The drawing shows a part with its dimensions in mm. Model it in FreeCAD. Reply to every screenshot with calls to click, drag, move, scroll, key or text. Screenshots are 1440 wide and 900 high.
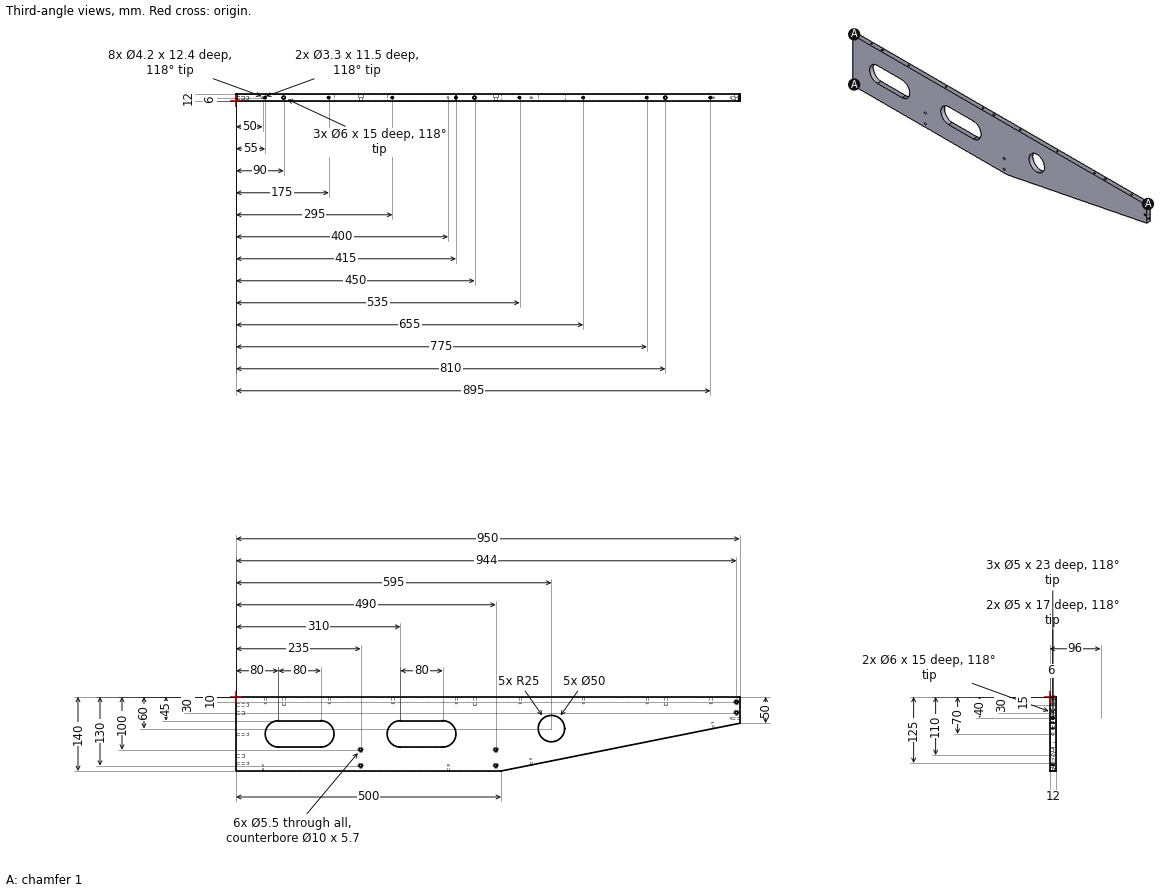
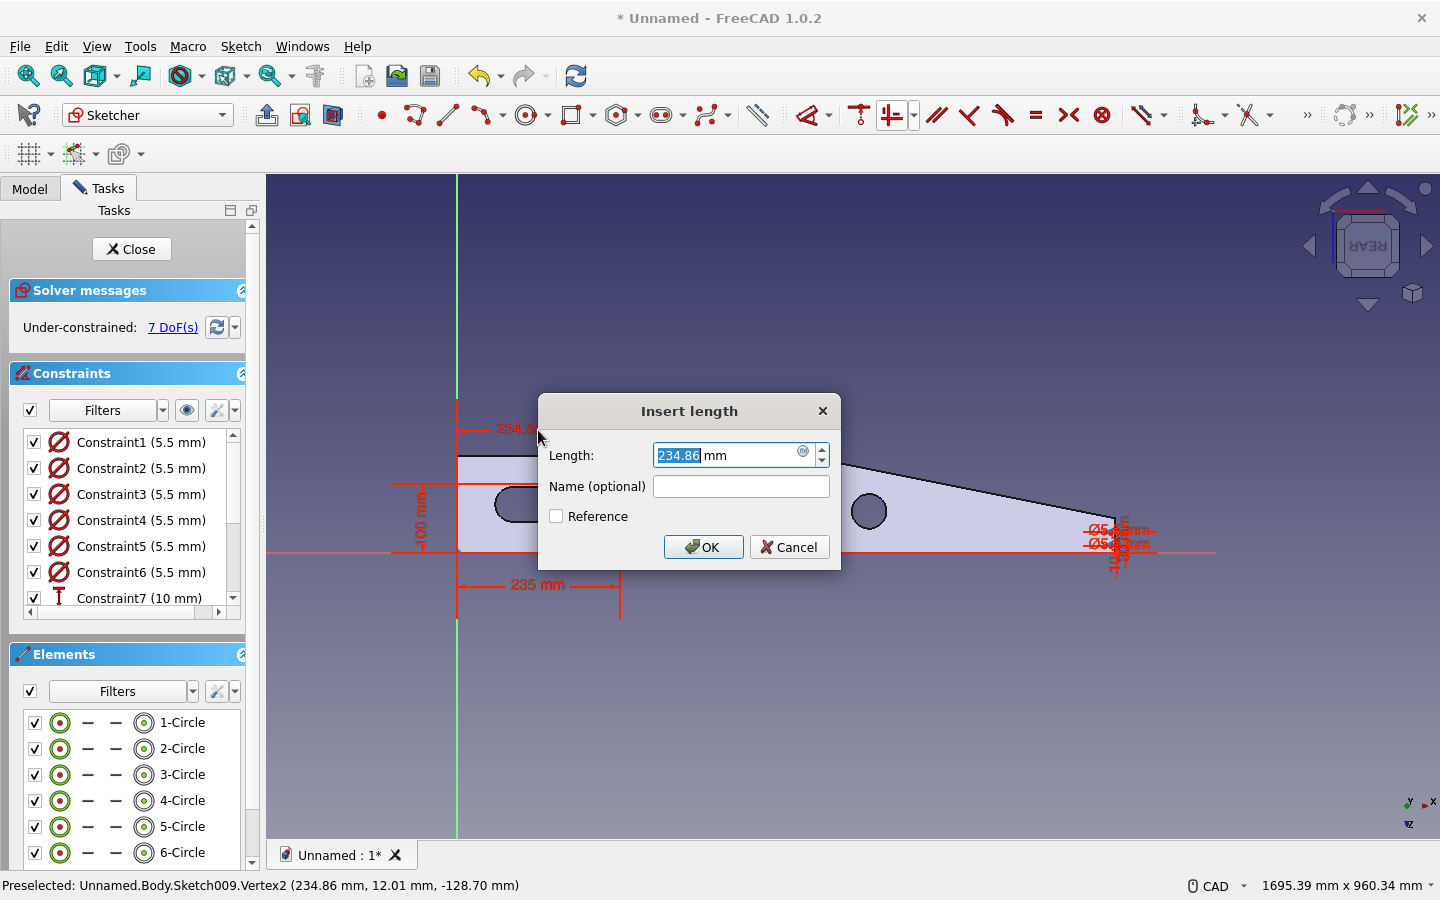
text(235)
key(Return)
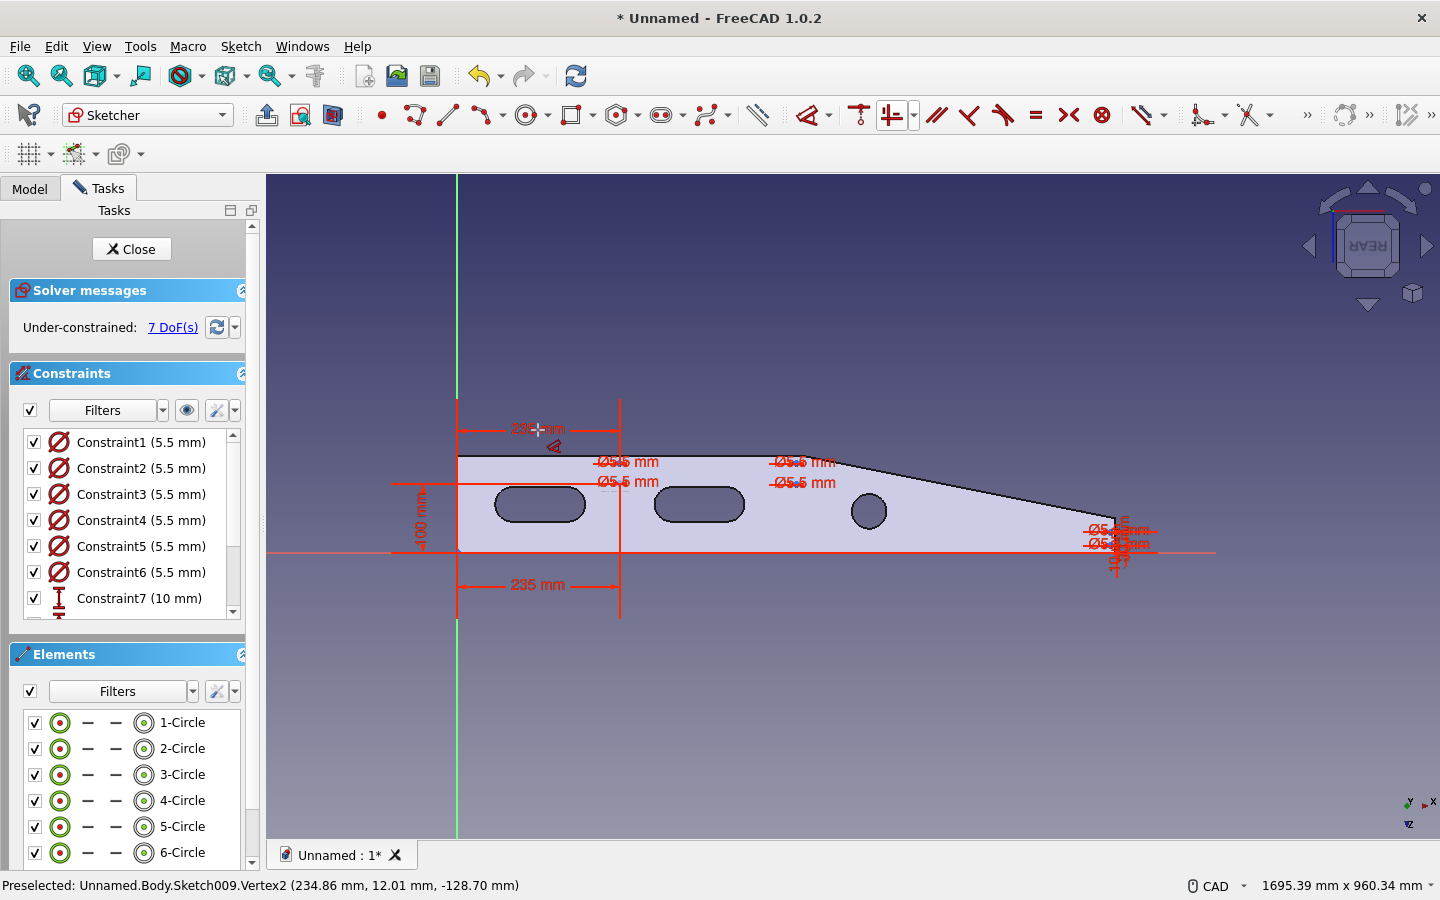
click(620, 464)
click(423, 488)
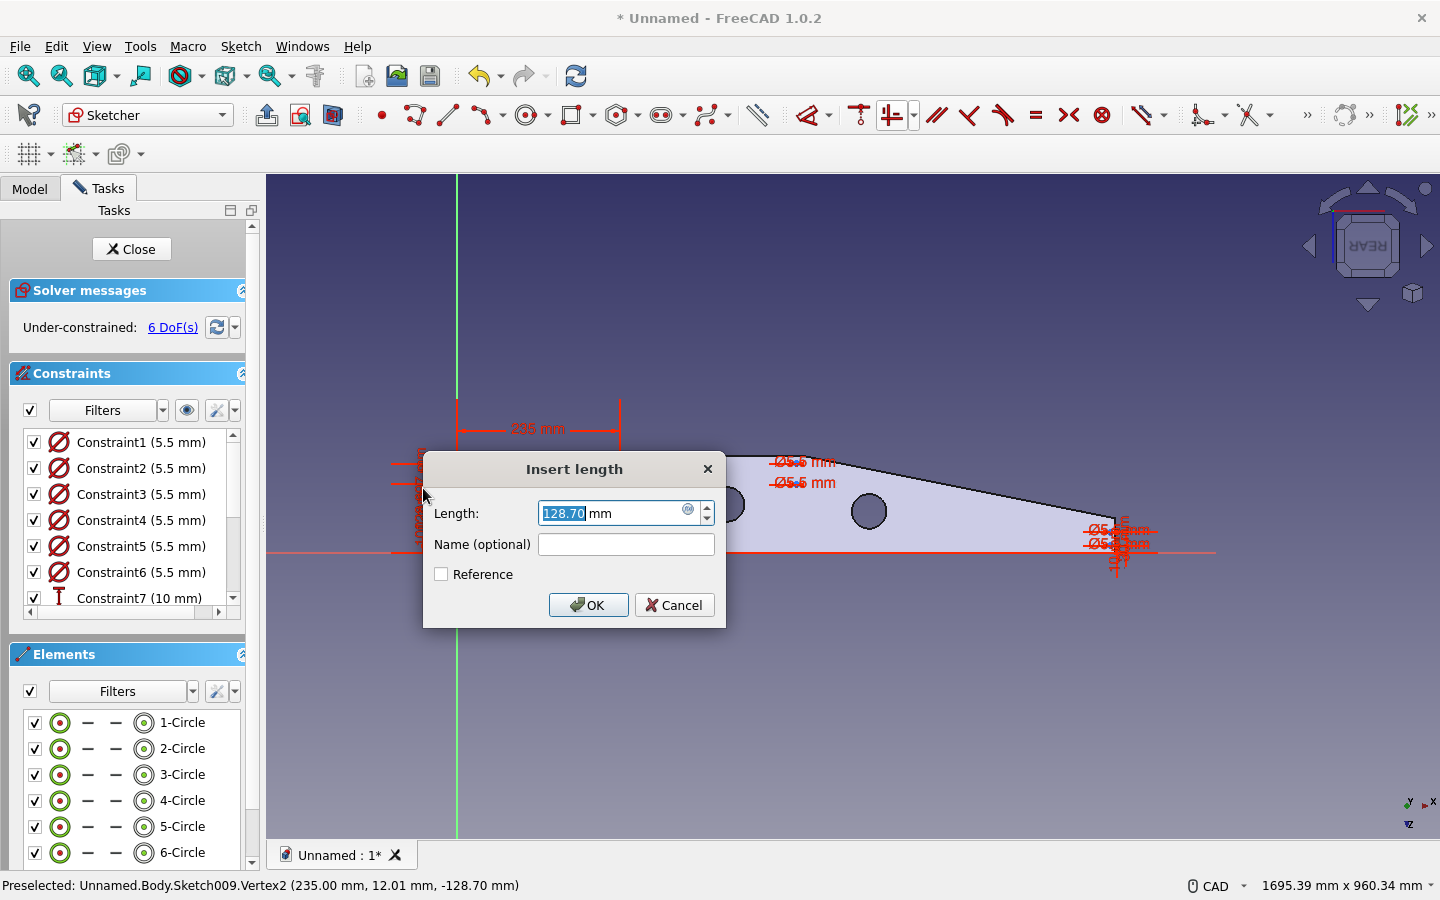
text(130)
key(Return)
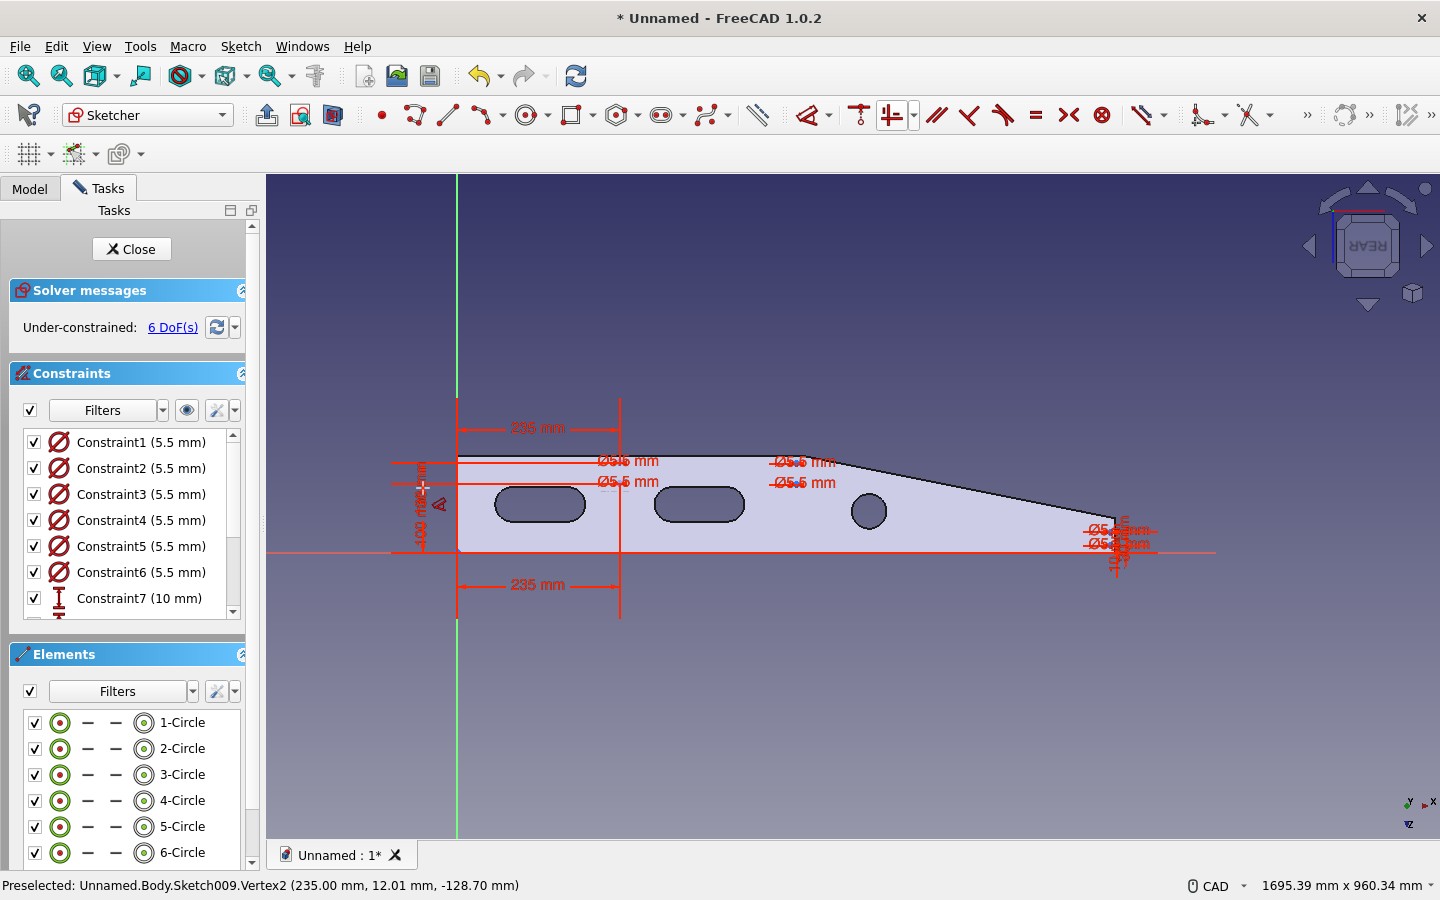
click(797, 485)
click(627, 587)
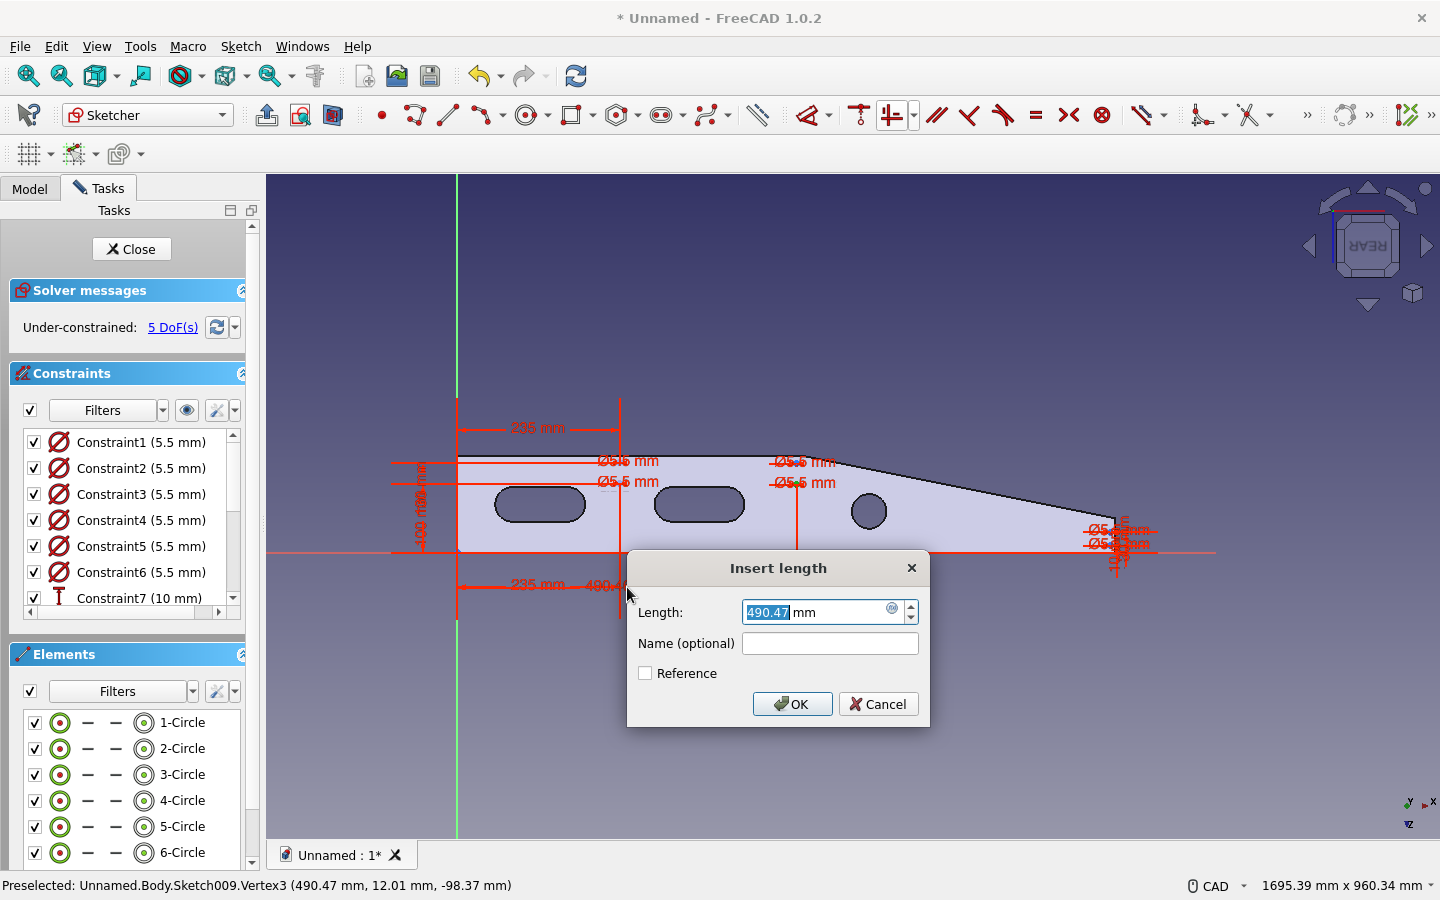
text(490)
key(Return)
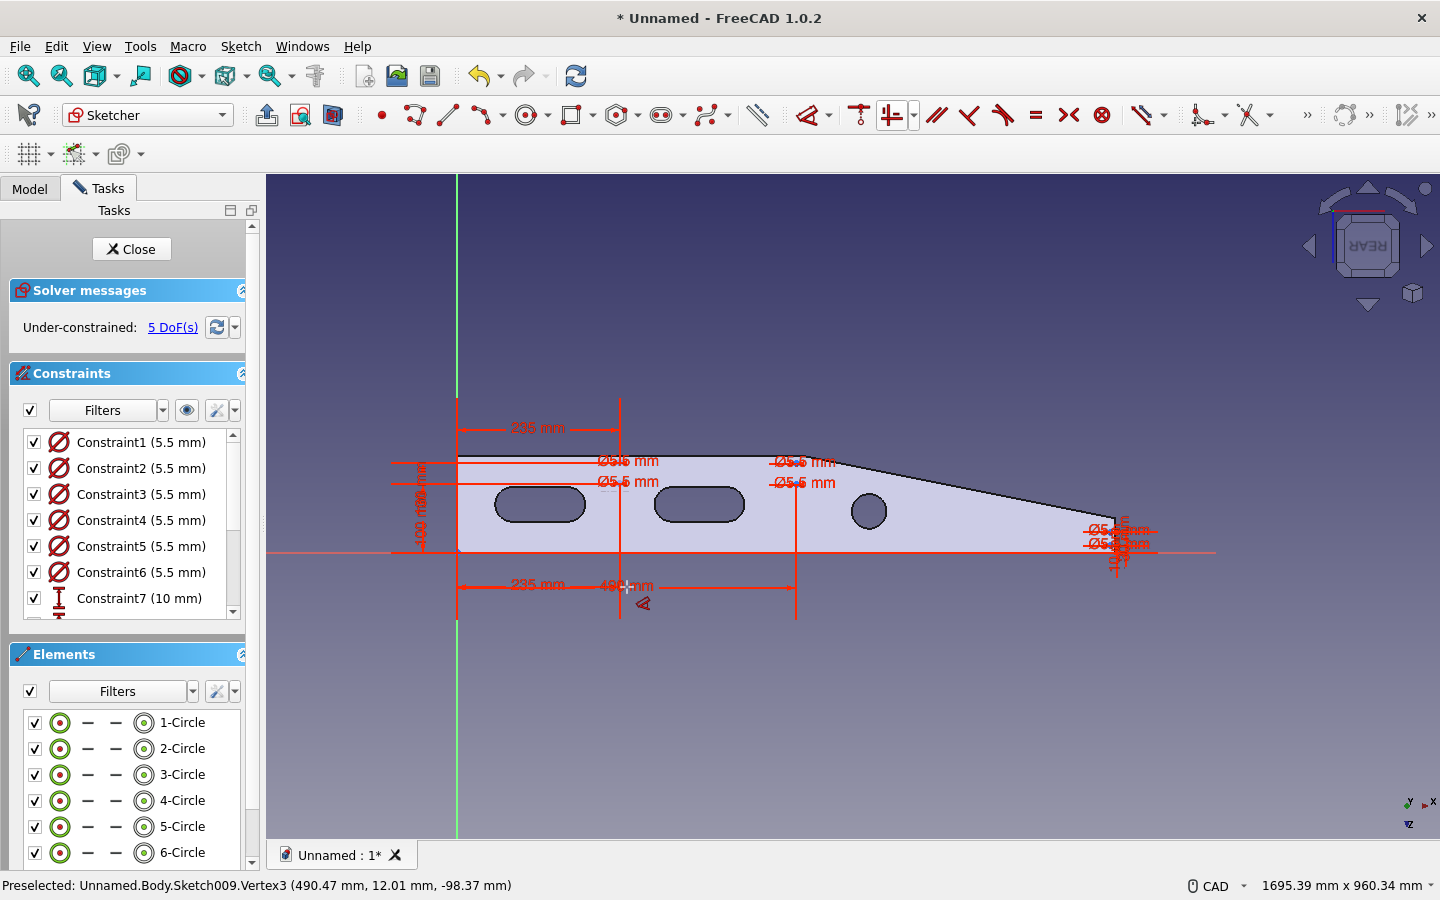
click(796, 485)
click(830, 519)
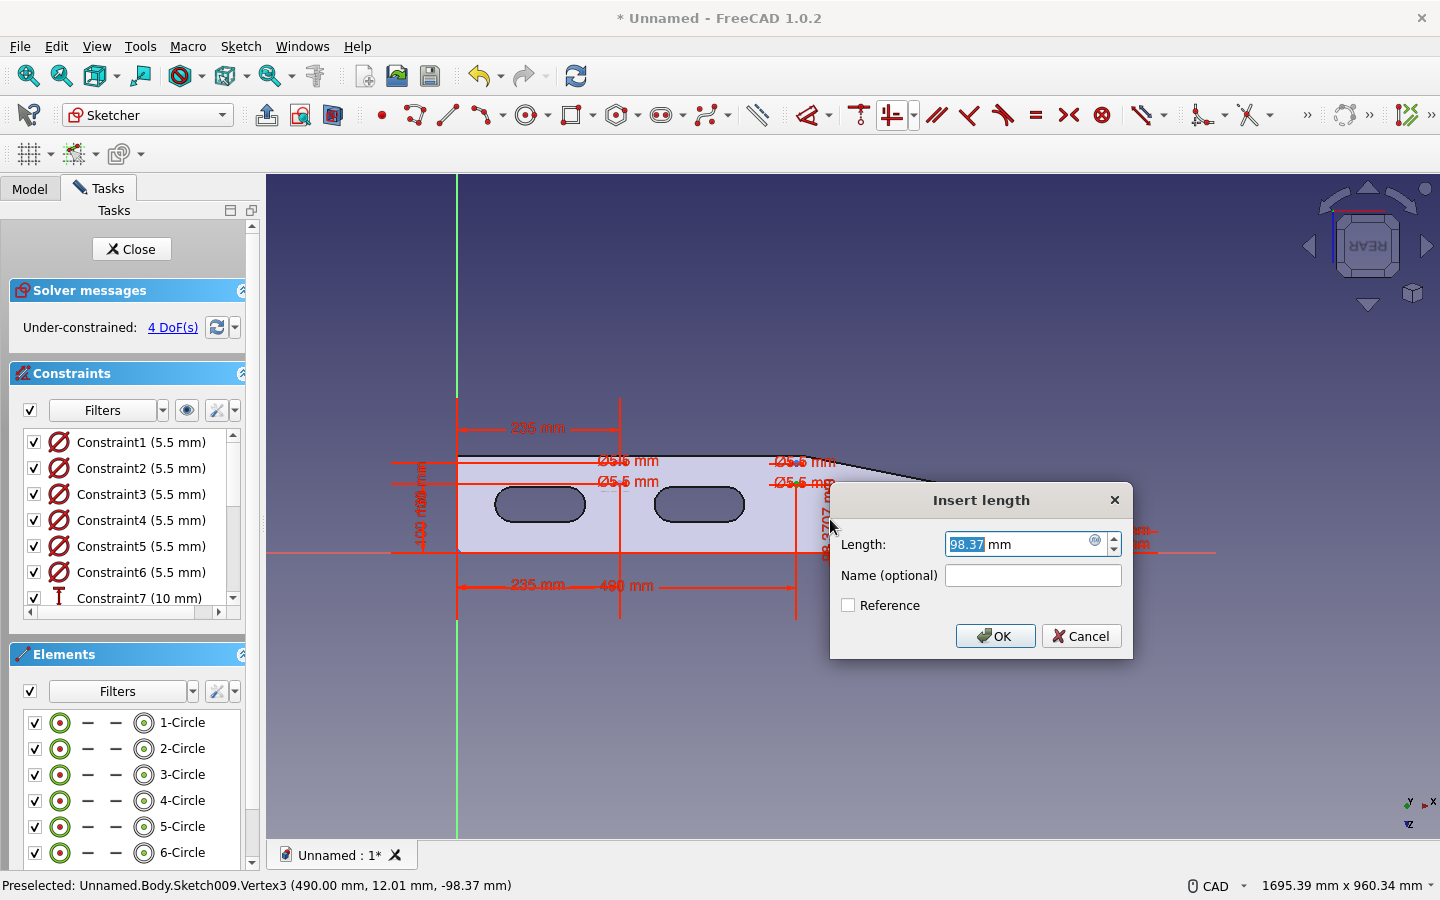
text(100)
key(Return)